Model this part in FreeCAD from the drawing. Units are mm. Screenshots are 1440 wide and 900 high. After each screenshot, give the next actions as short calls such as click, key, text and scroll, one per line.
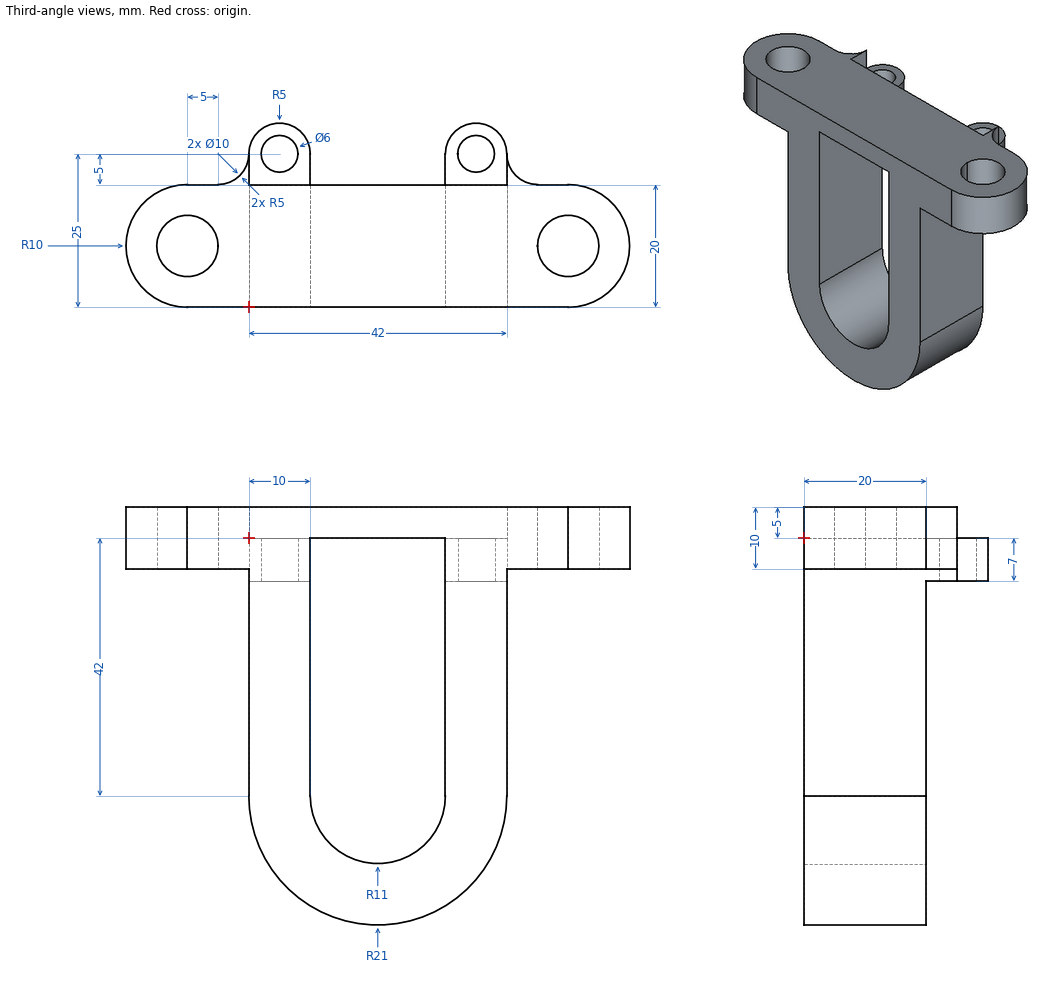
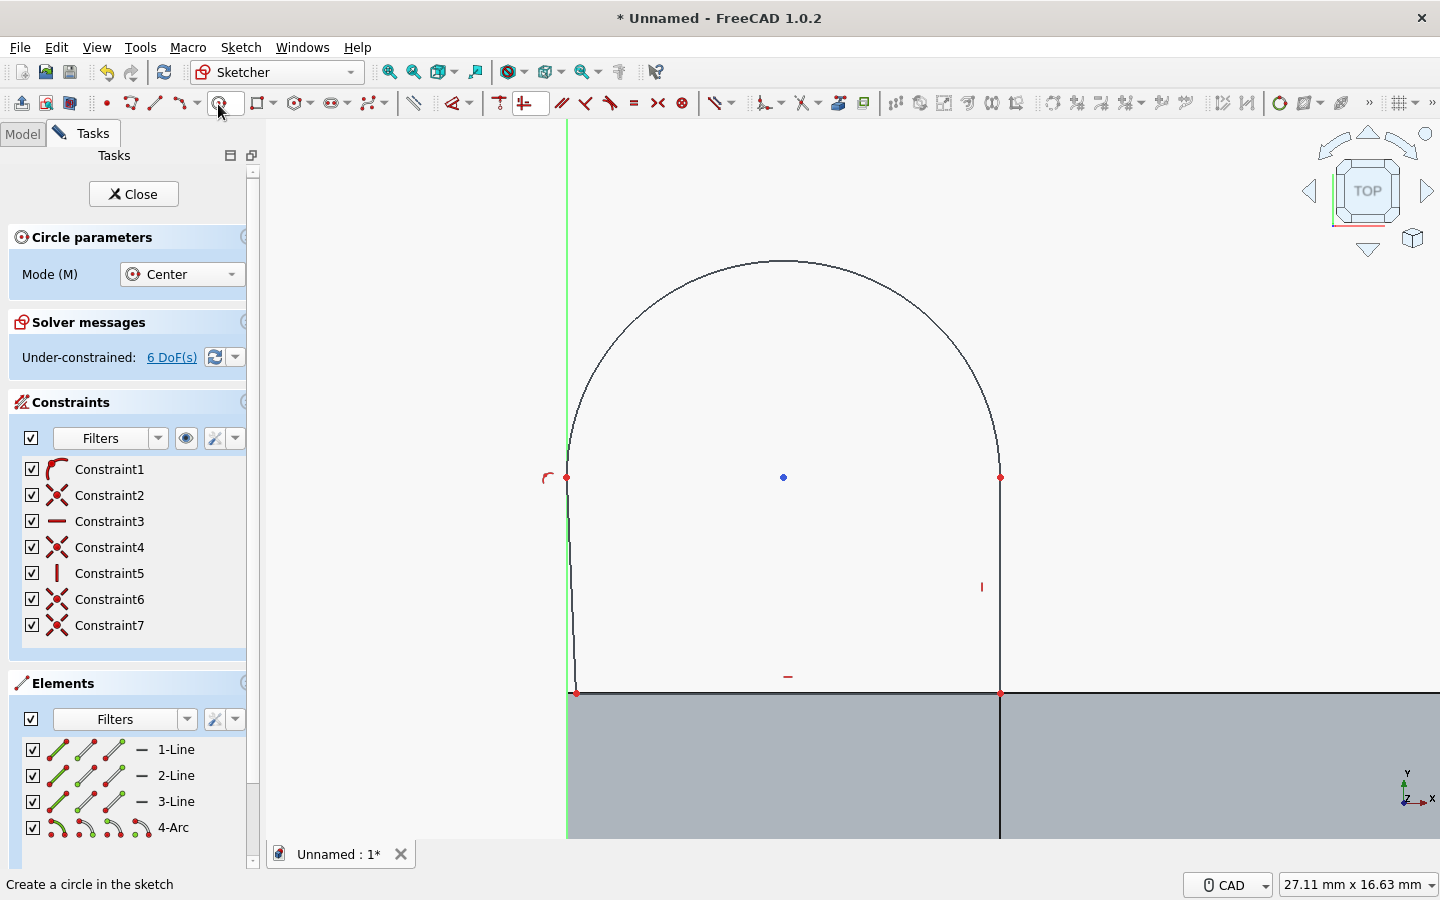
click(783, 477)
click(875, 385)
key(Escape)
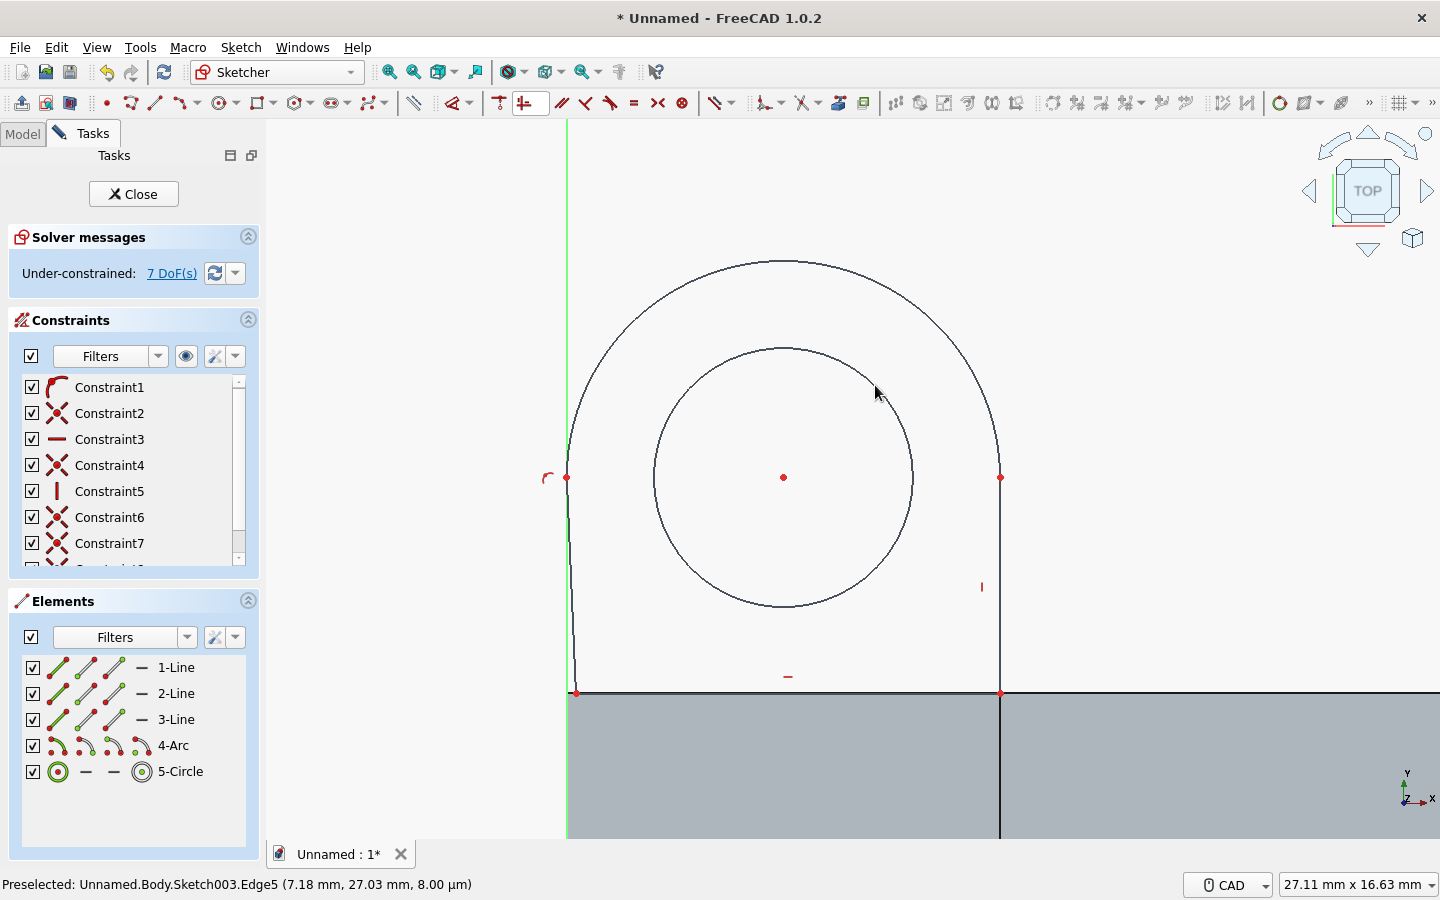
click(570, 543)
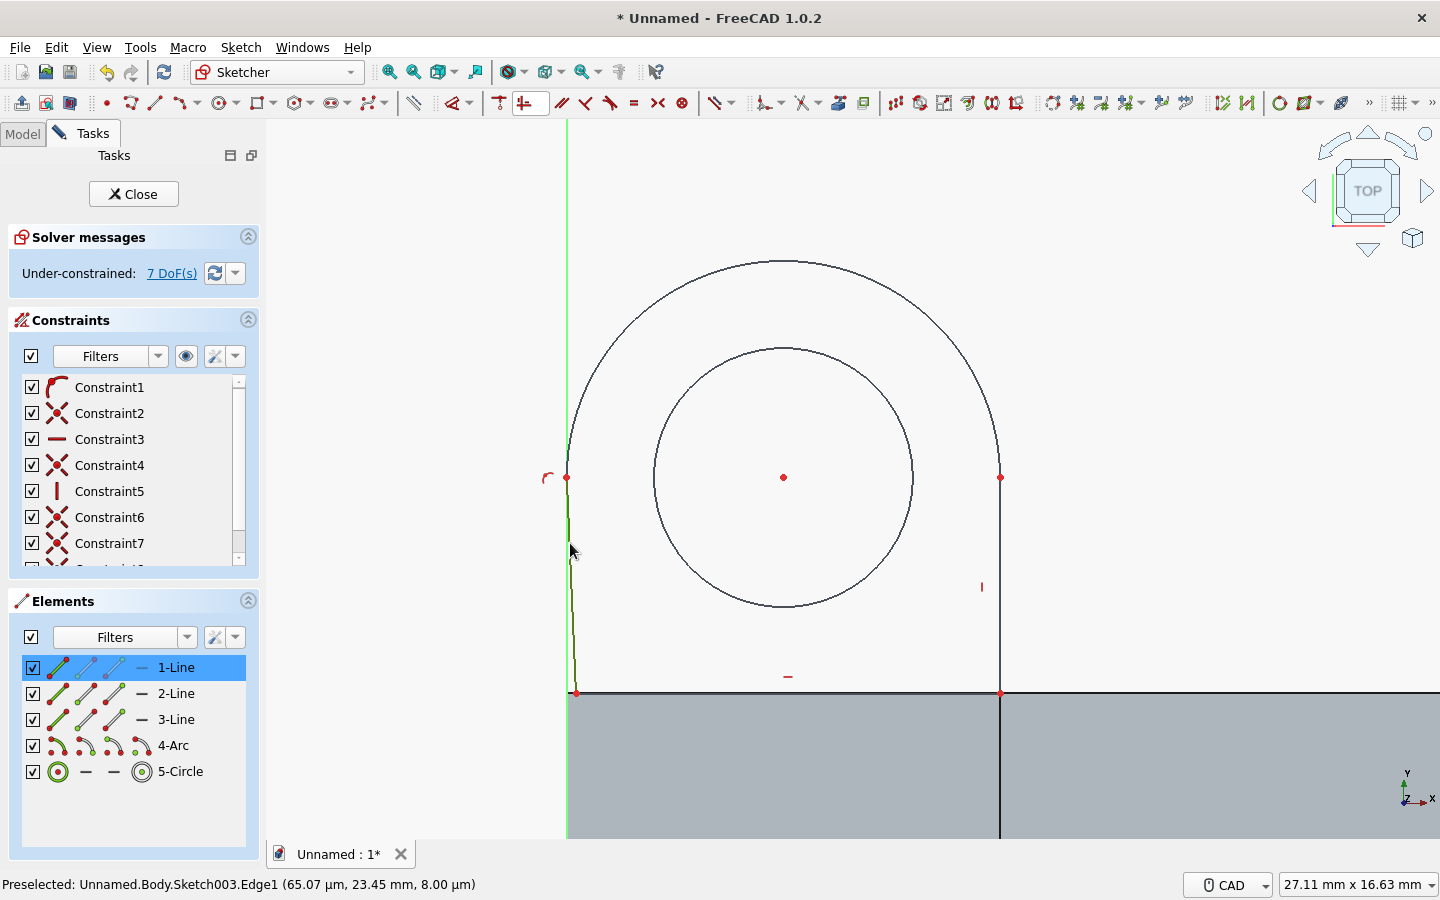
click(911, 302)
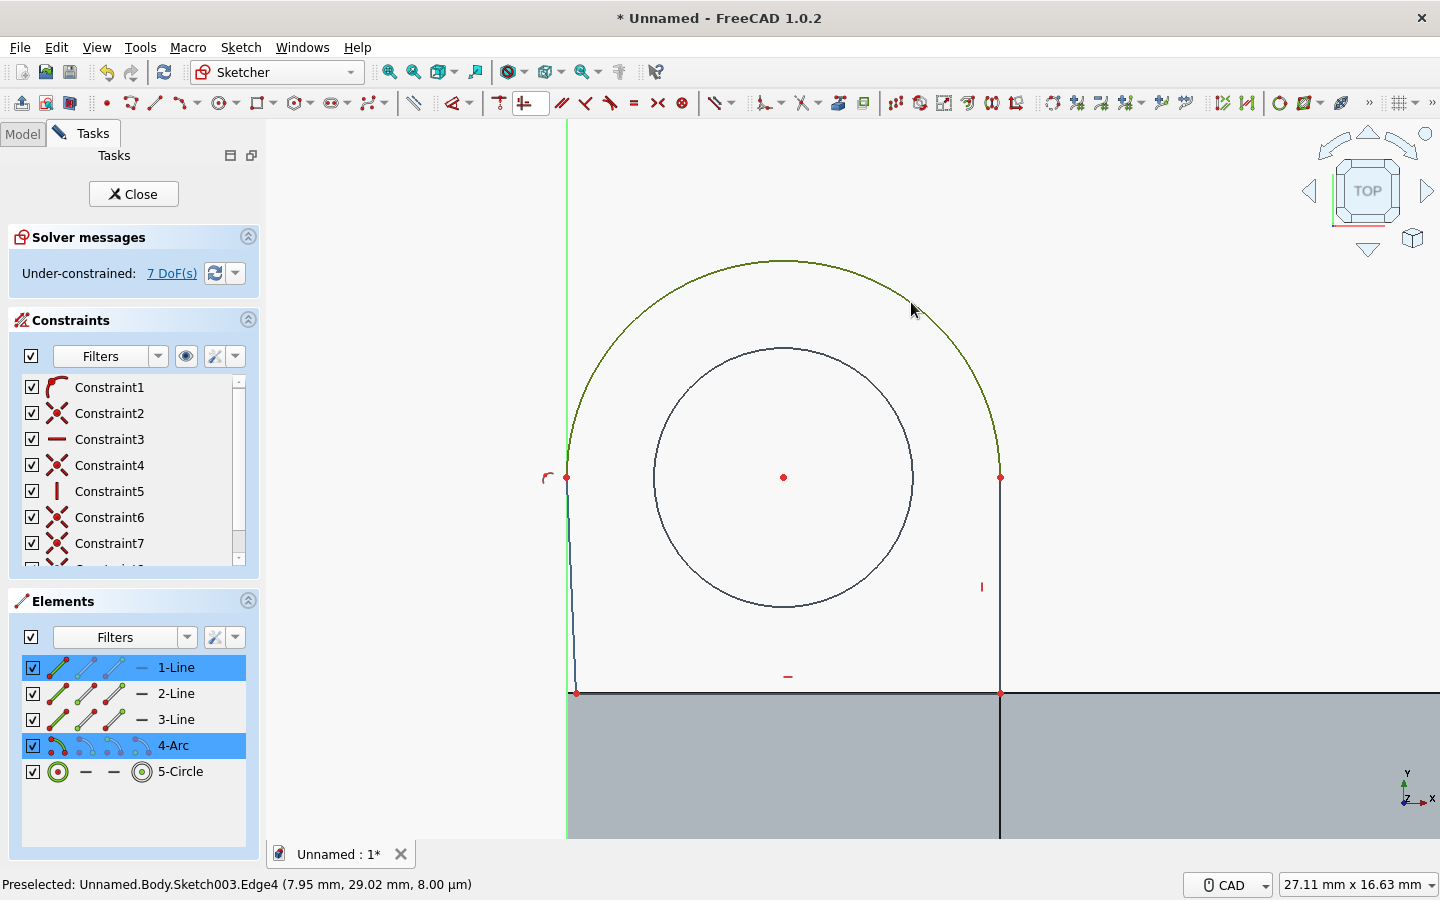
click(610, 104)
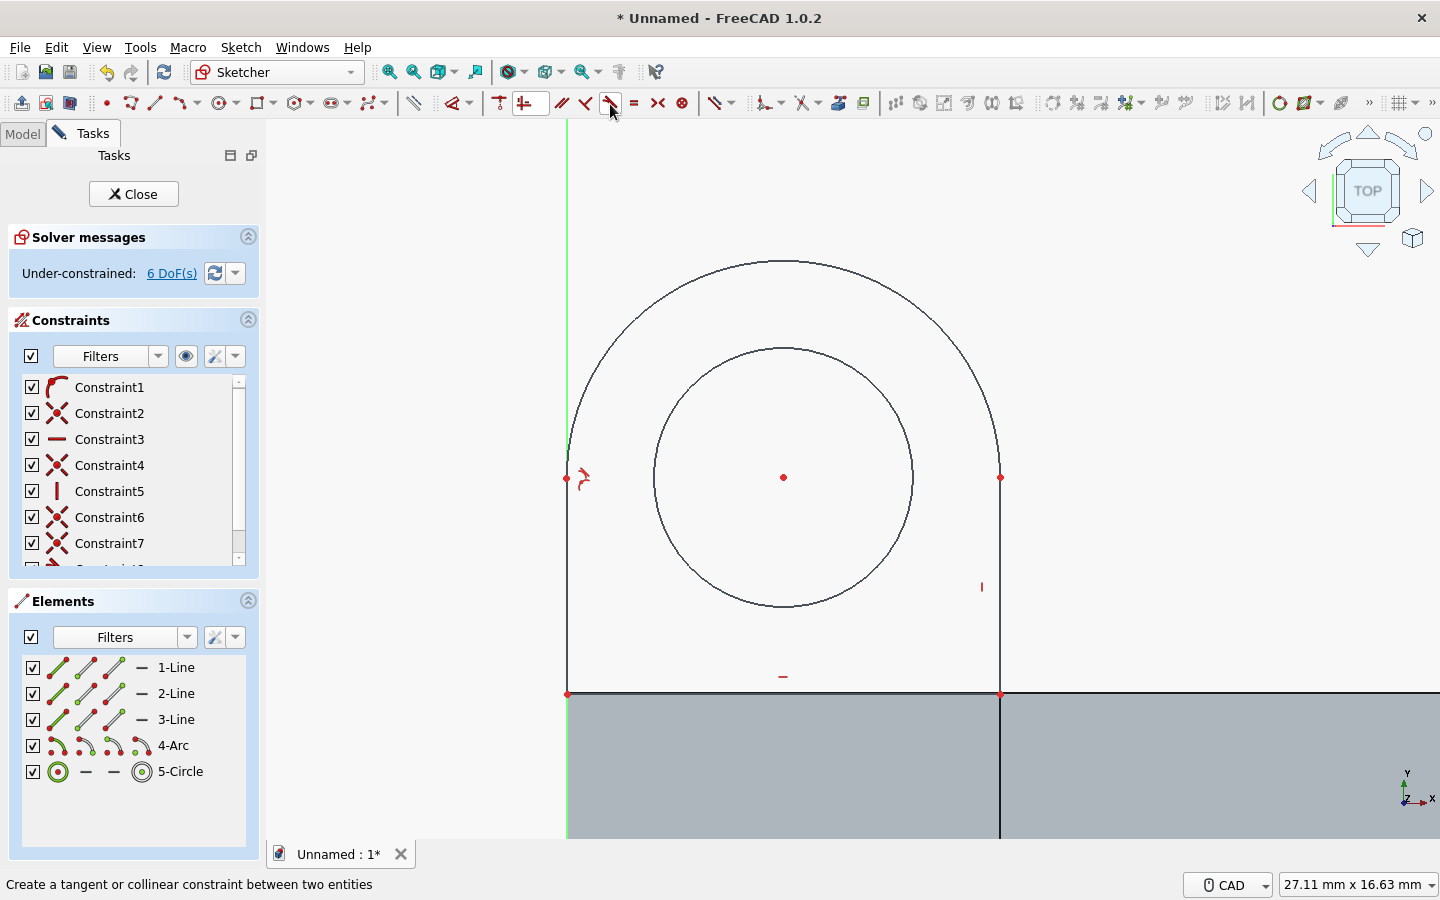
click(1000, 629)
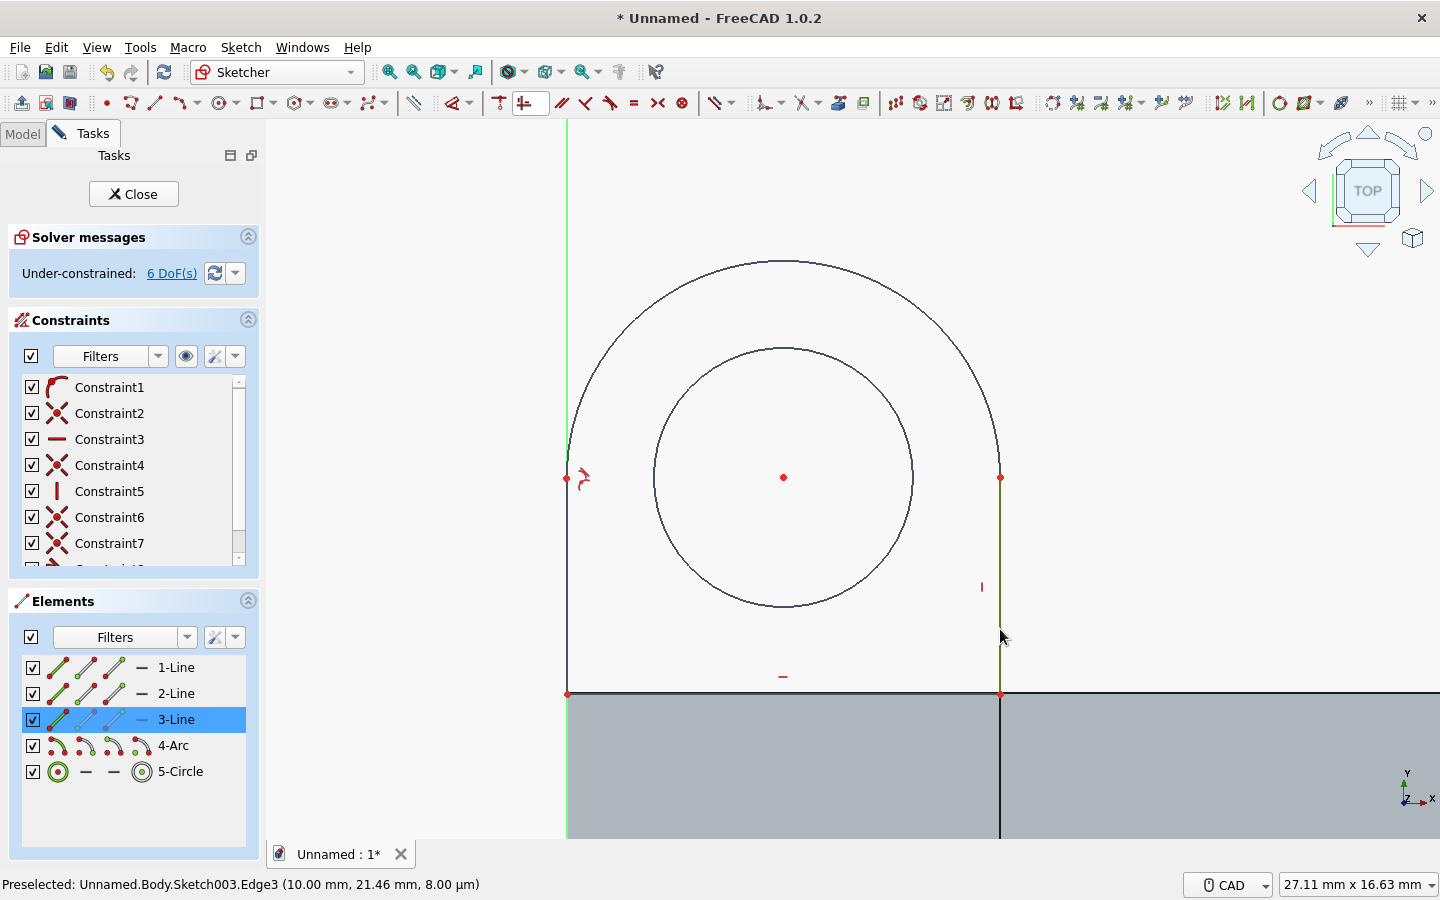
click(911, 302)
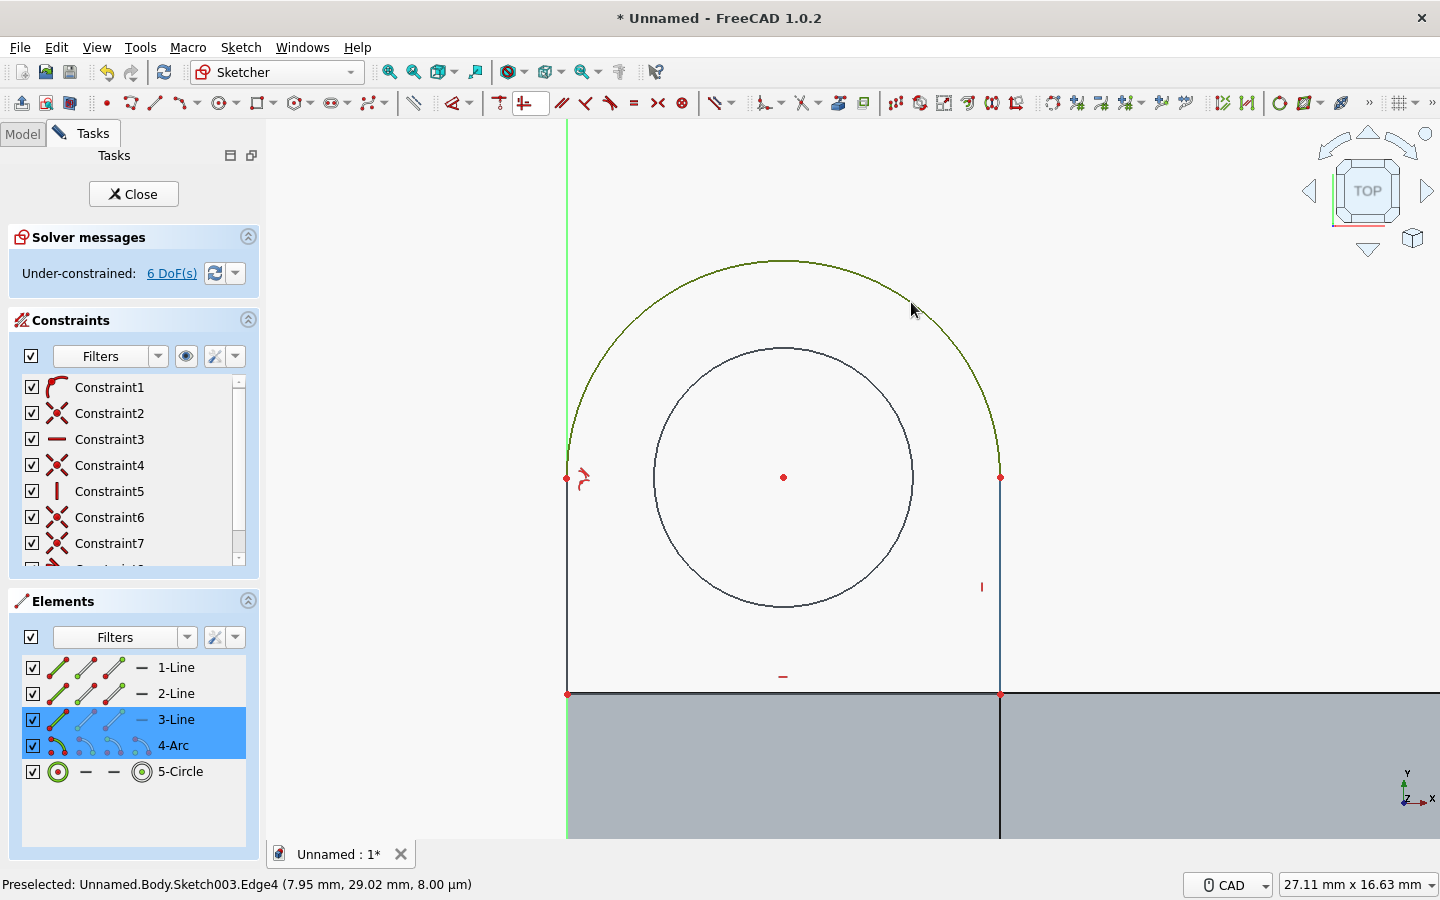
click(610, 104)